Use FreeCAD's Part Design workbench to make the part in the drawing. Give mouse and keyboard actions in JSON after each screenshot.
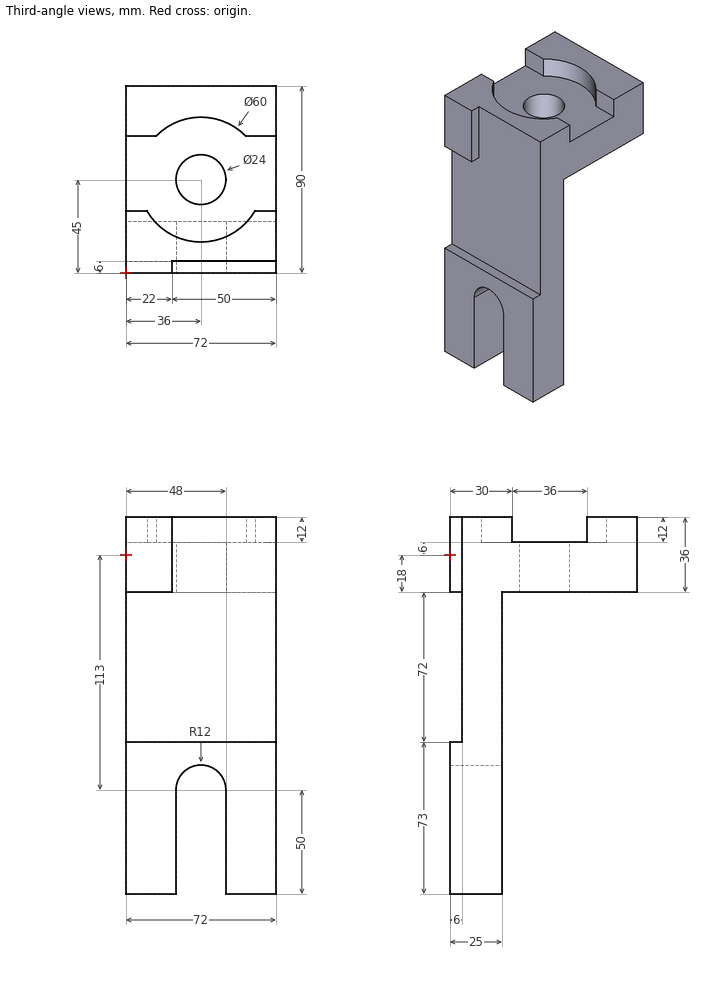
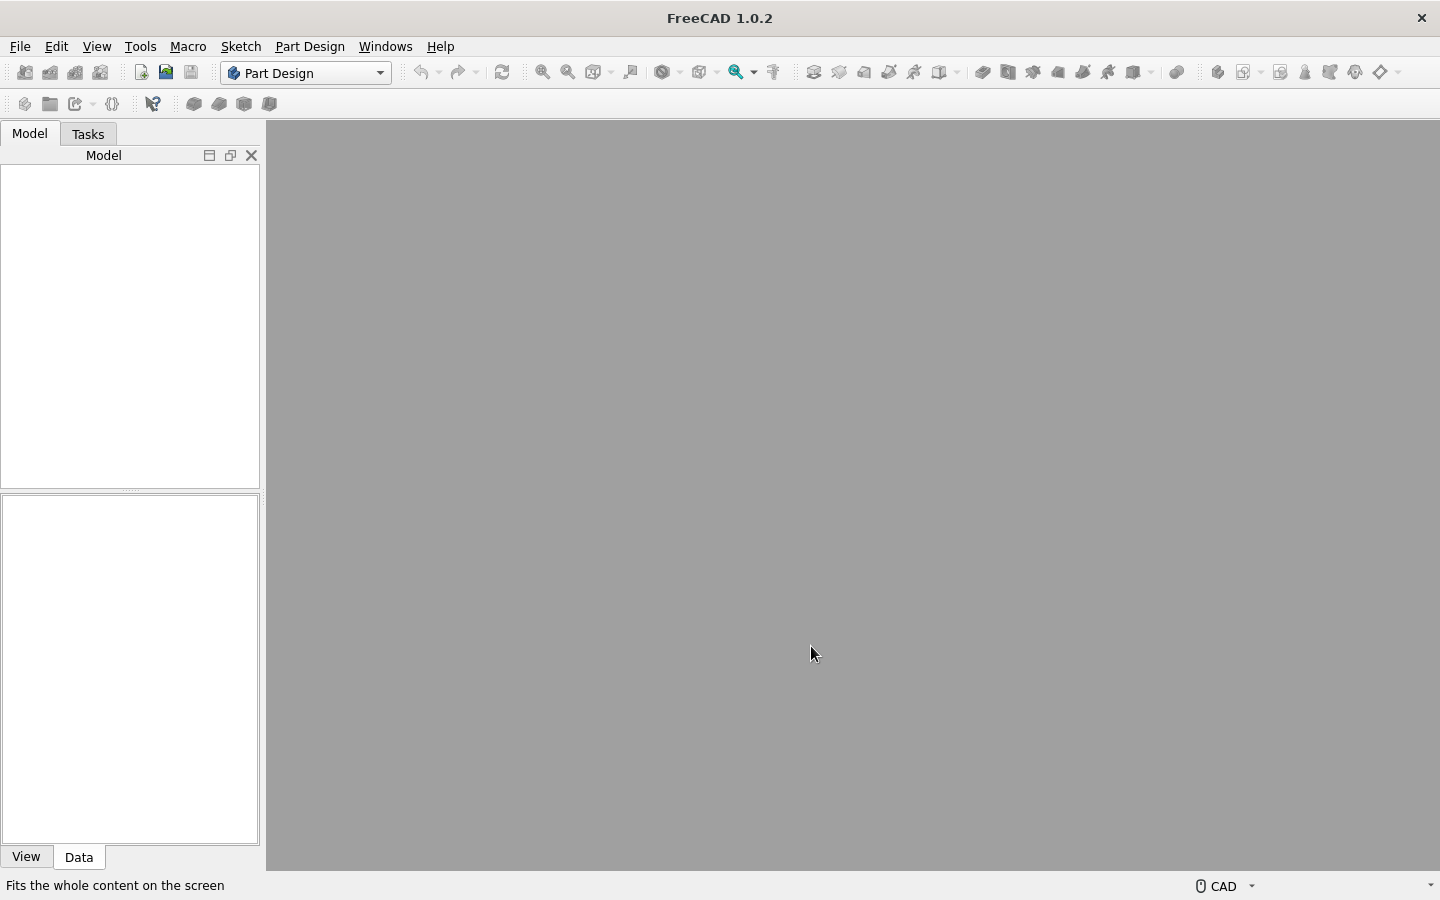
{"action": "key", "text": "ctrl+n"}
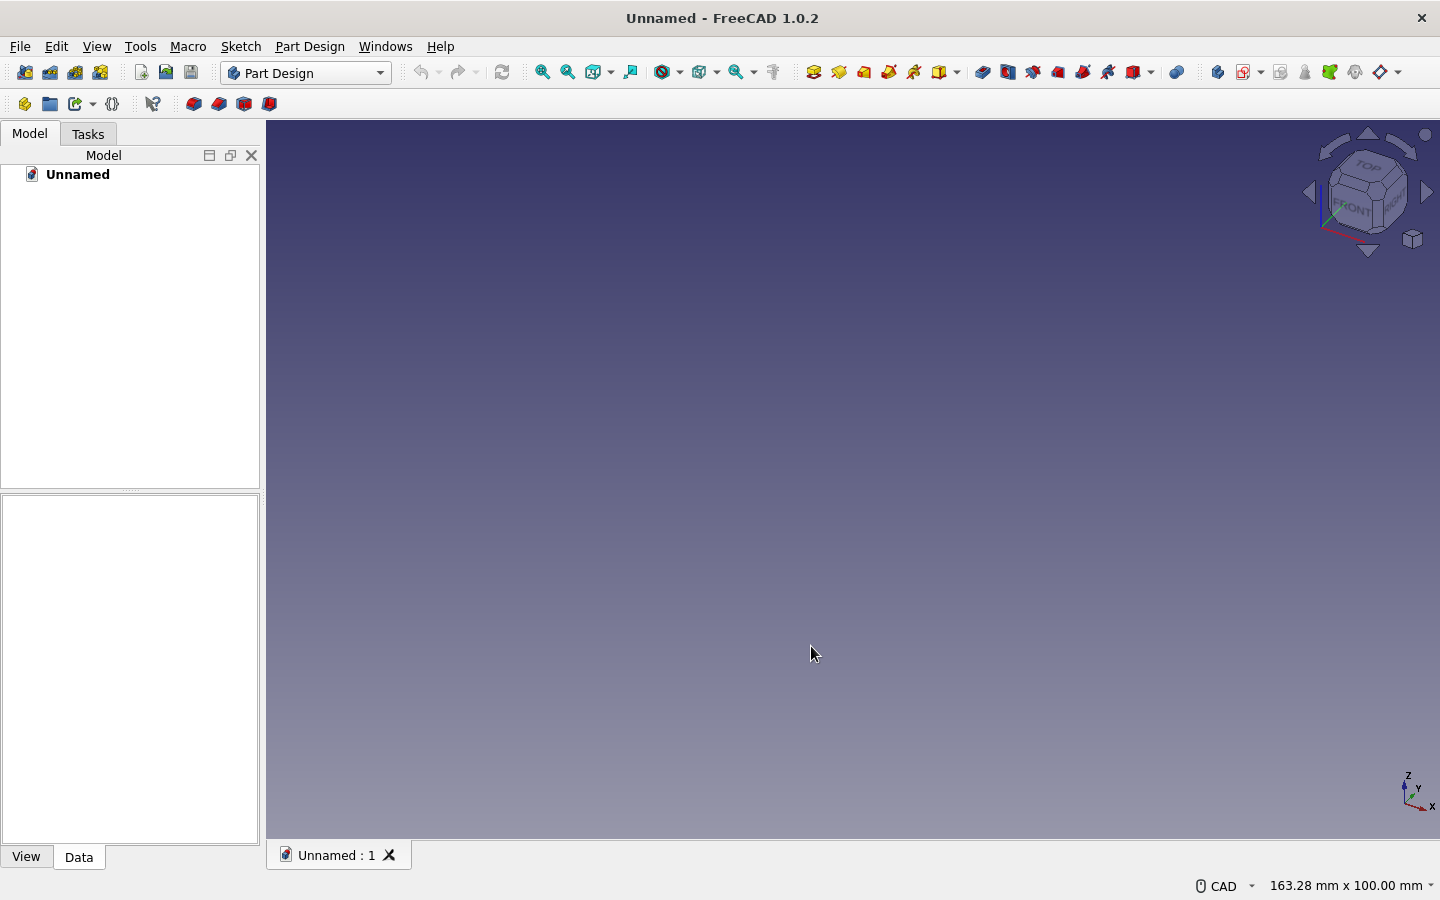
{"action": "left_click", "coordinate": [1242, 72]}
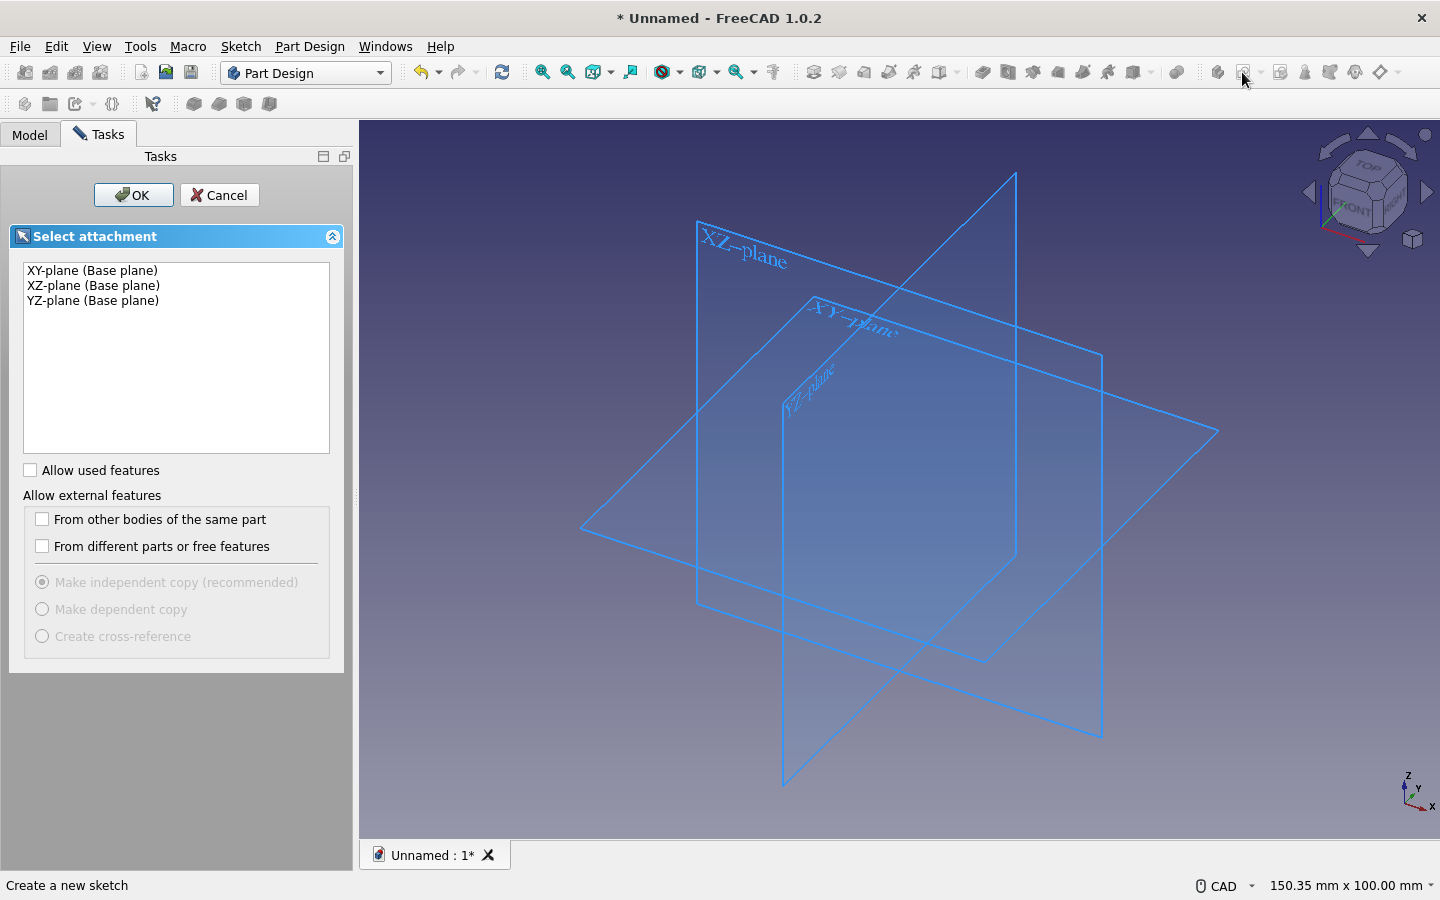
{"action": "left_click", "coordinate": [84, 270]}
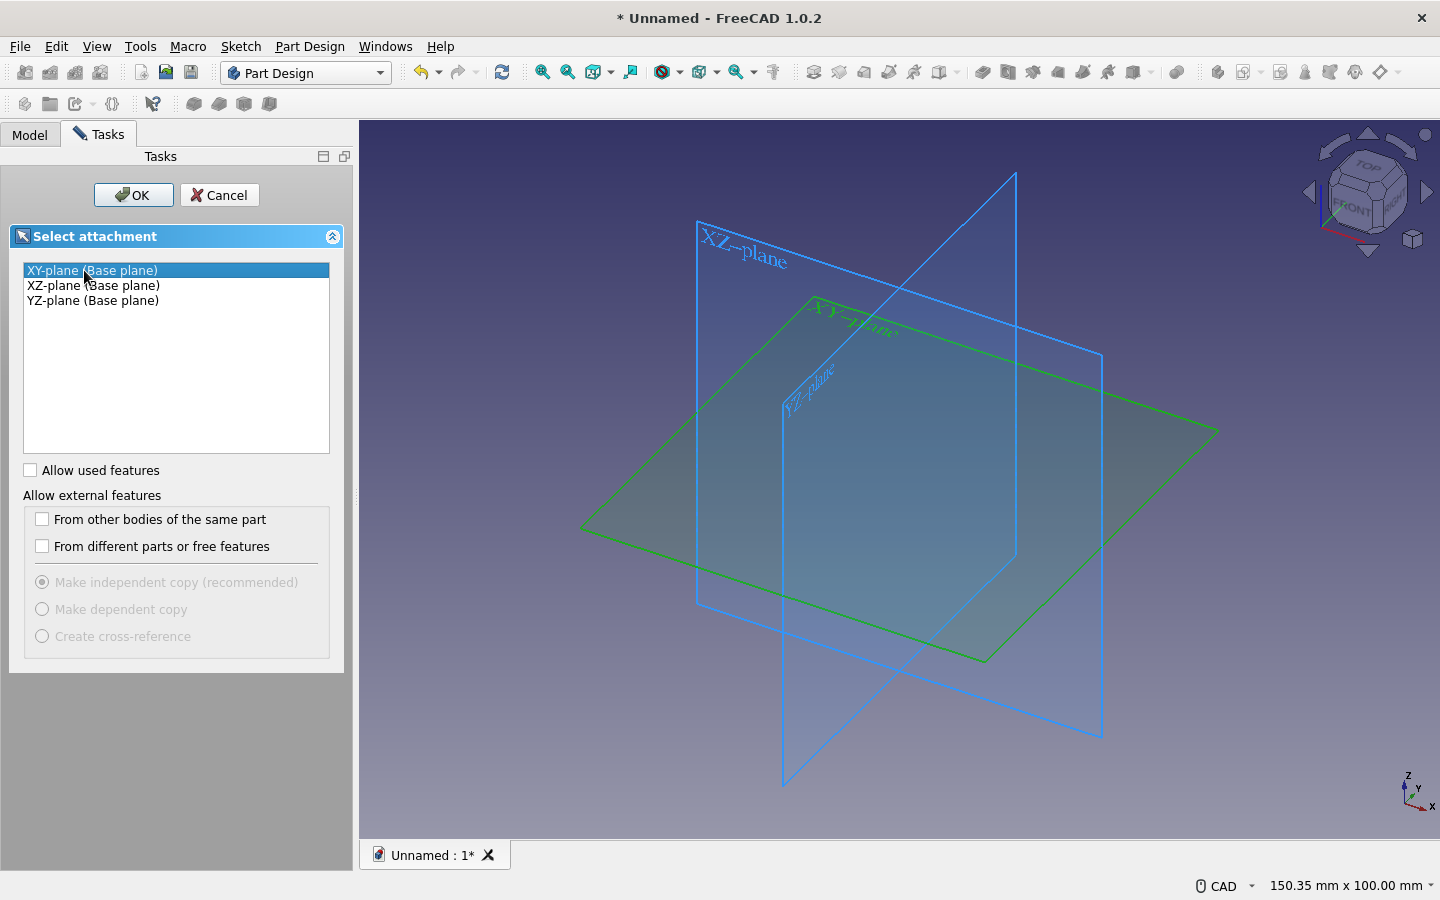
{"action": "left_click", "coordinate": [134, 195]}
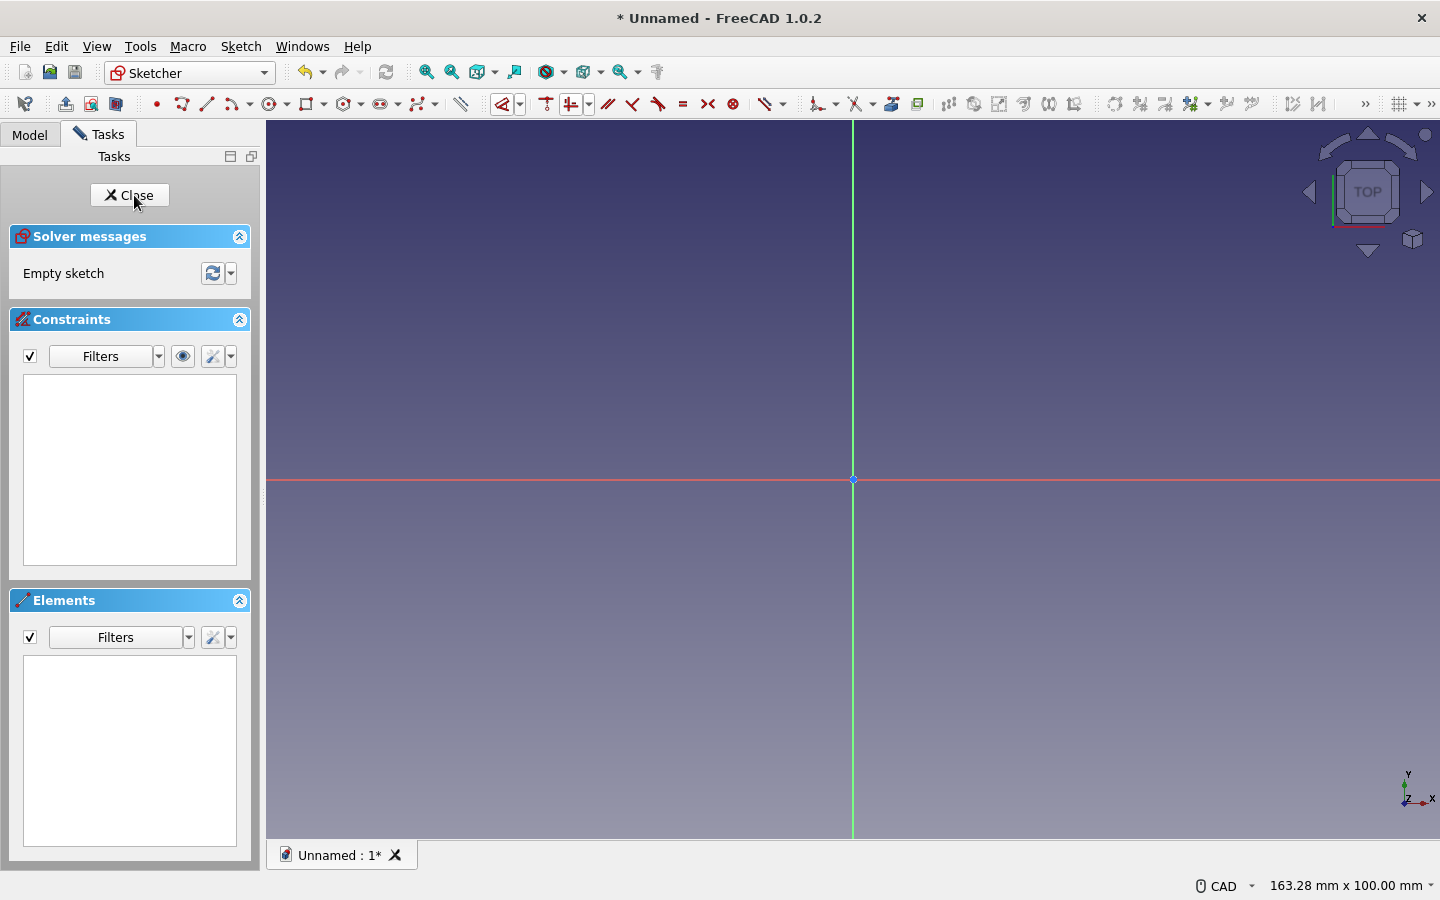
{"action": "scroll", "coordinate": [386, 811], "scroll_direction": "down", "scroll_amount": 3}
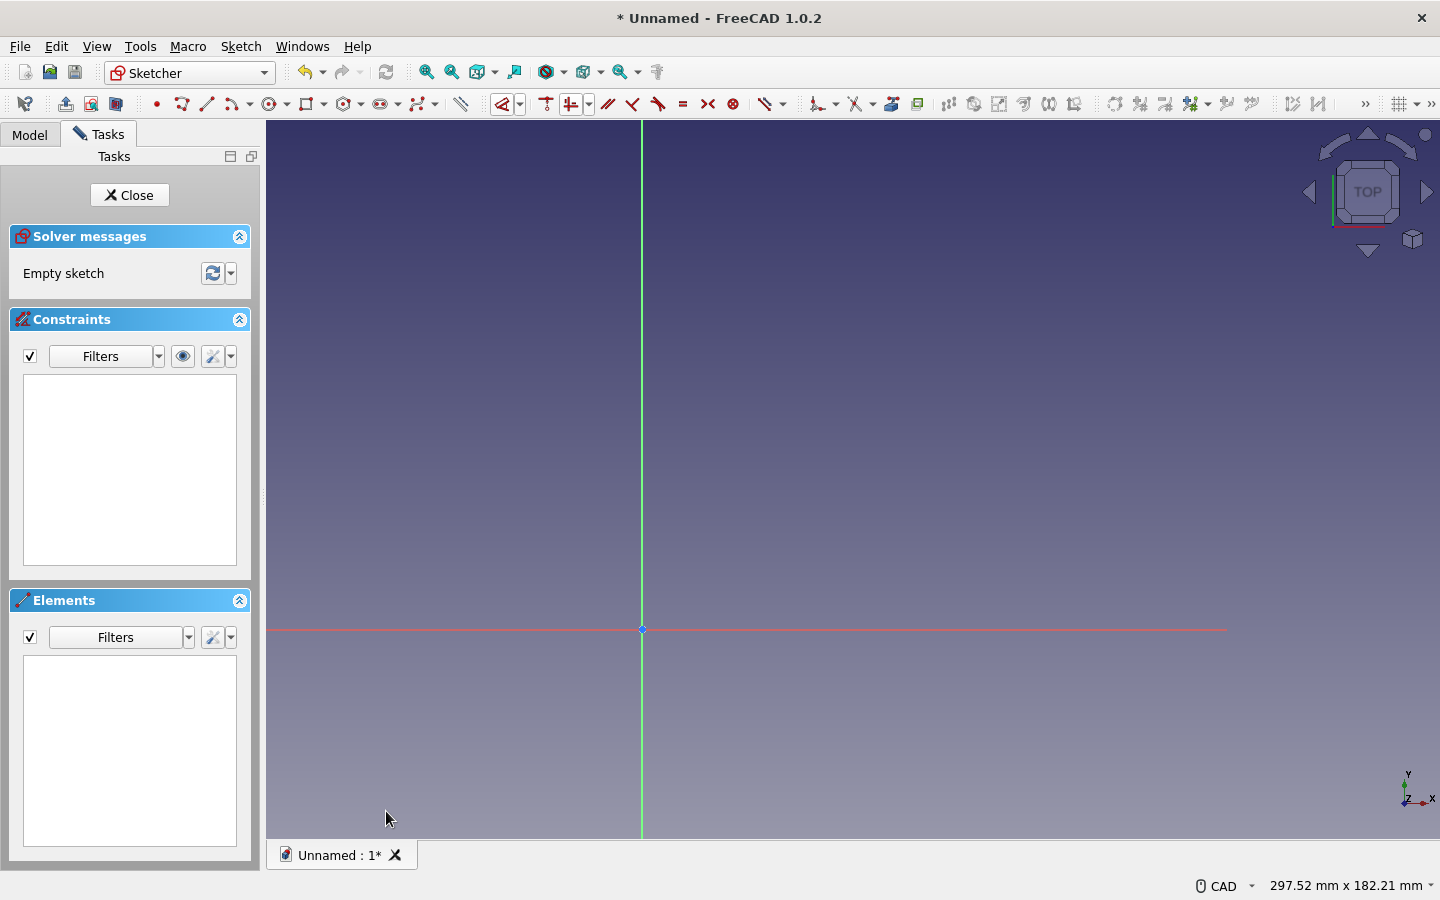
{"action": "key", "text": "g r"}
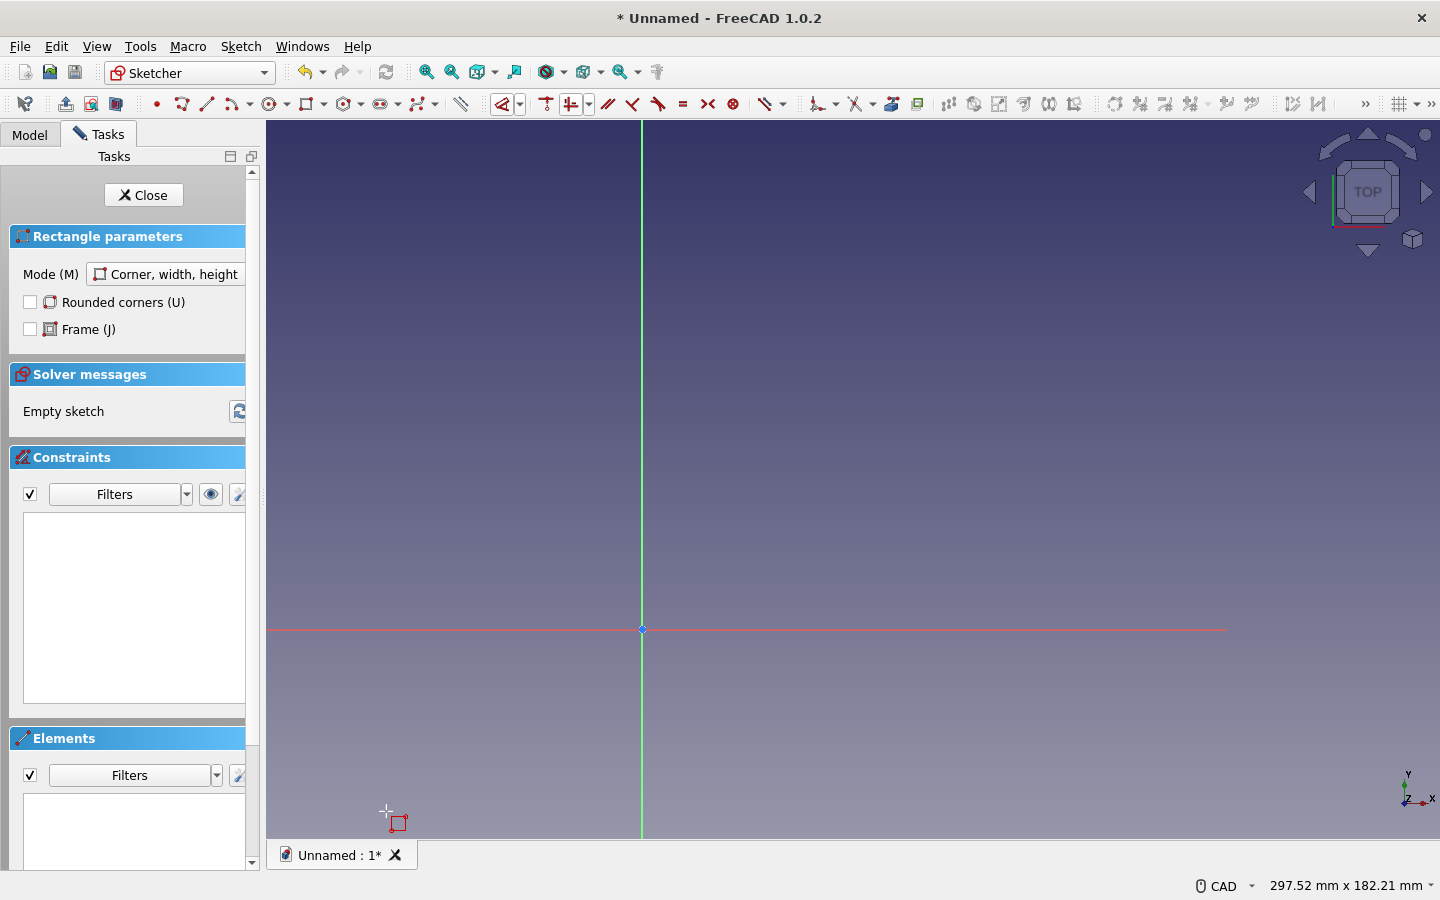
{"action": "left_click", "coordinate": [642, 630]}
{"action": "mouse_move", "coordinate": [926, 274]}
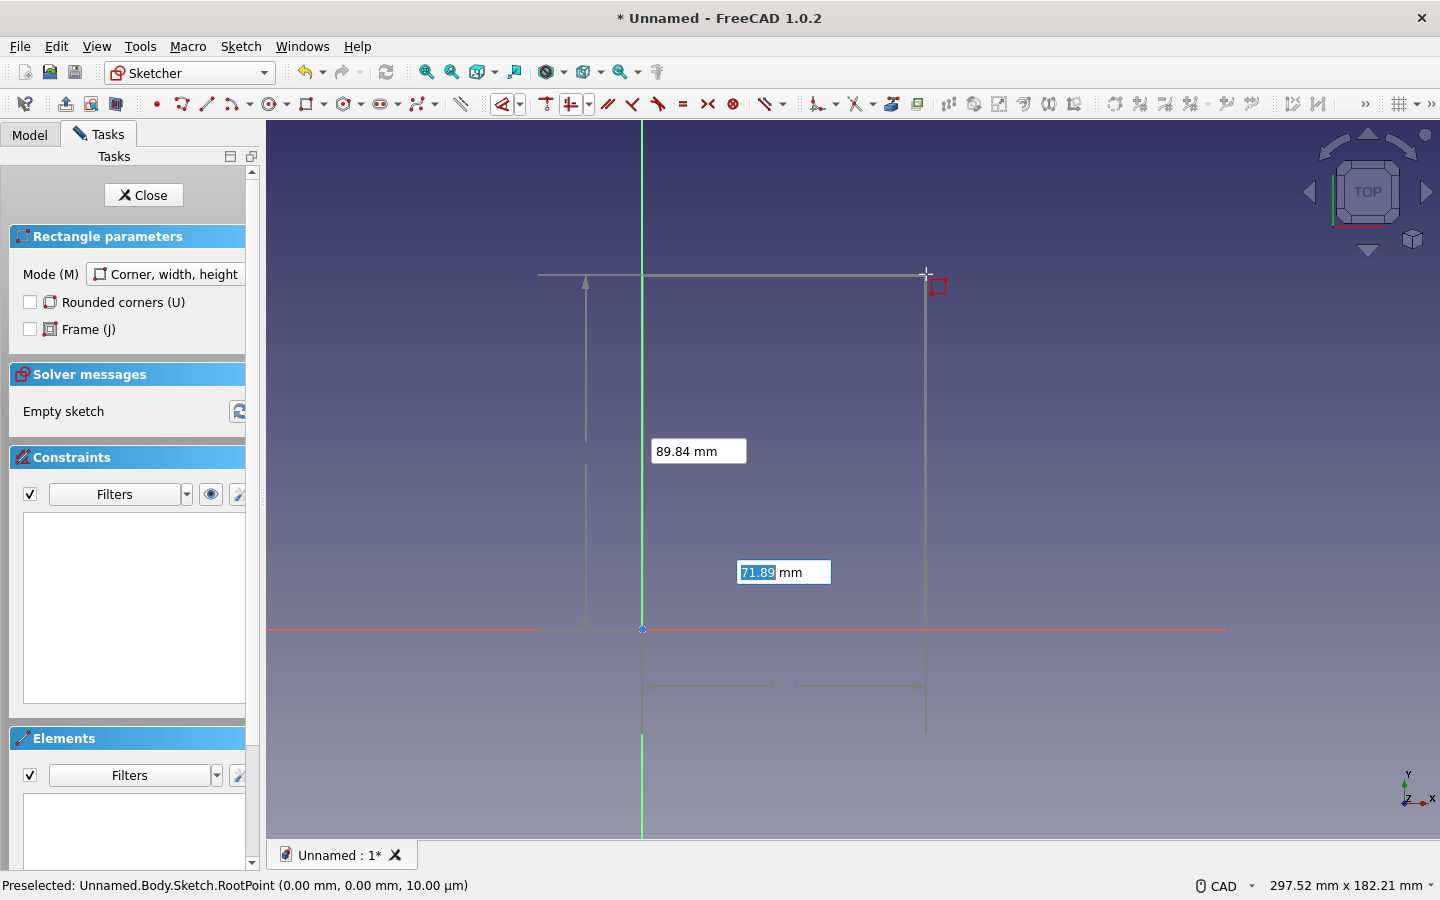
{"action": "type", "text": "72"}
{"action": "key", "text": "Tab"}
{"action": "type", "text": "90"}
{"action": "key", "text": "Return"}
{"action": "key", "text": "Escape"}